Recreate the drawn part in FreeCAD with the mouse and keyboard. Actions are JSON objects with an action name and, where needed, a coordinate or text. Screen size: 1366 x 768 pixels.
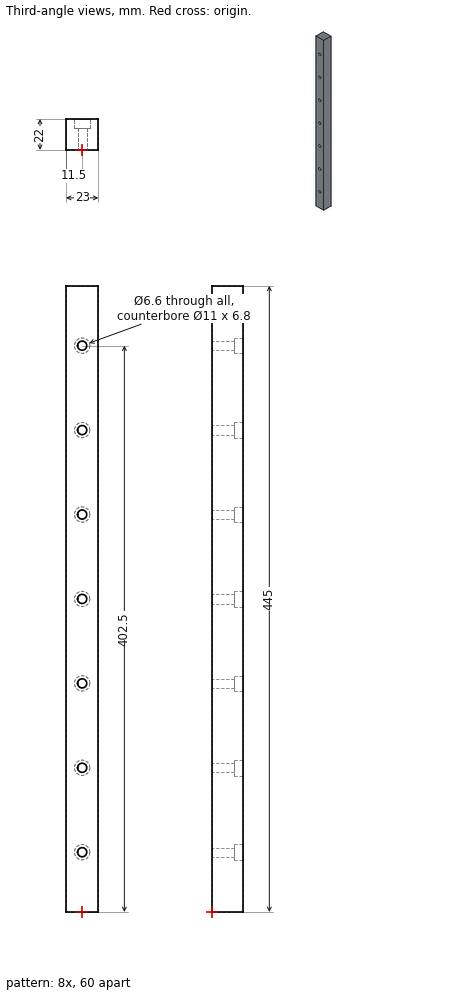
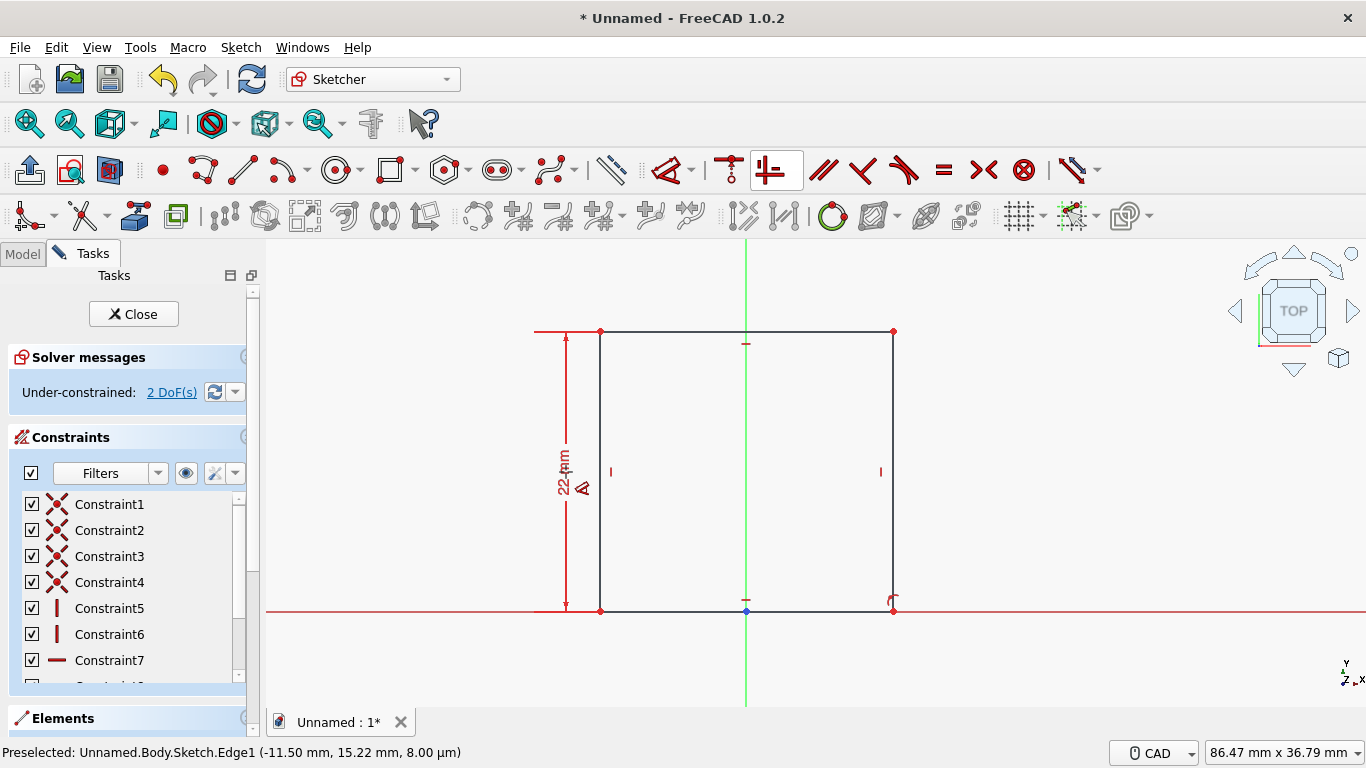
{"action": "left_click", "coordinate": [688, 612]}
{"action": "left_click", "coordinate": [679, 646]}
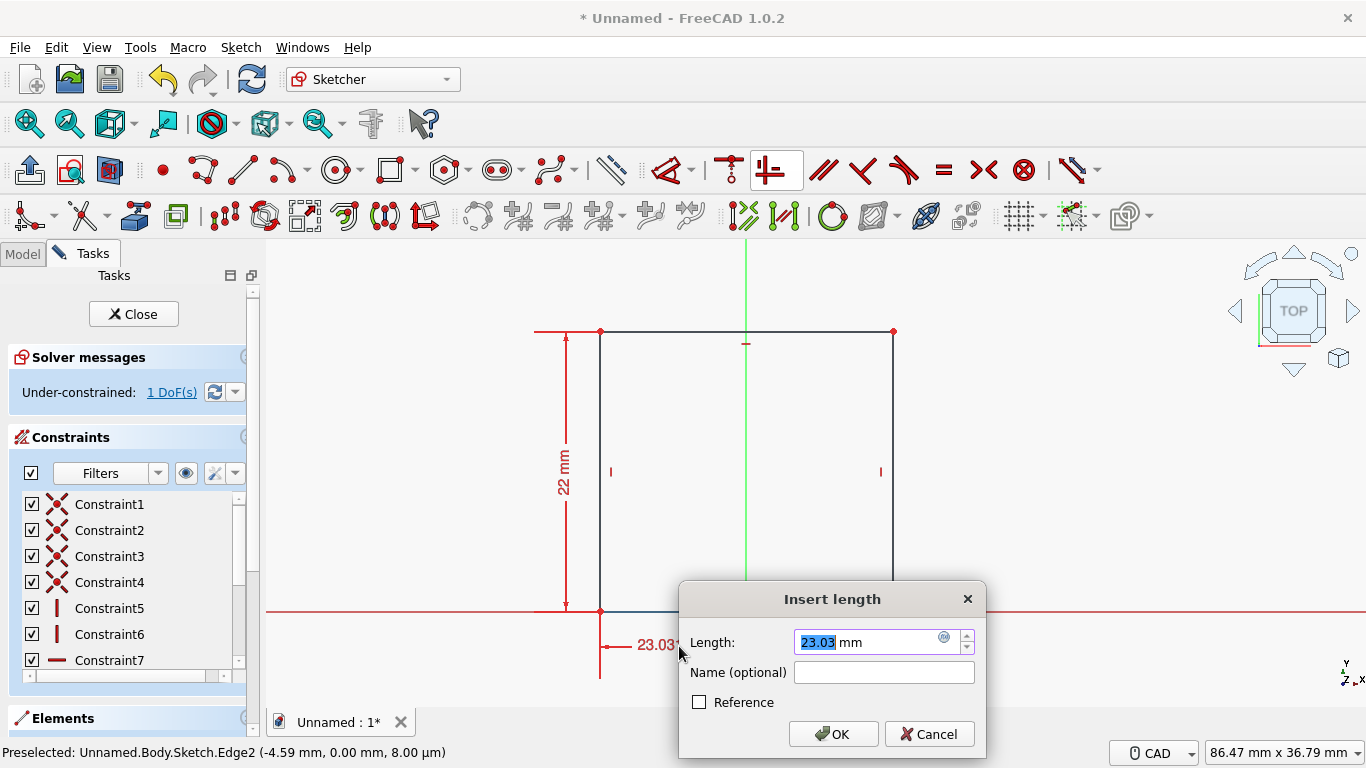
{"action": "type", "text": "23"}
{"action": "key", "text": "Return"}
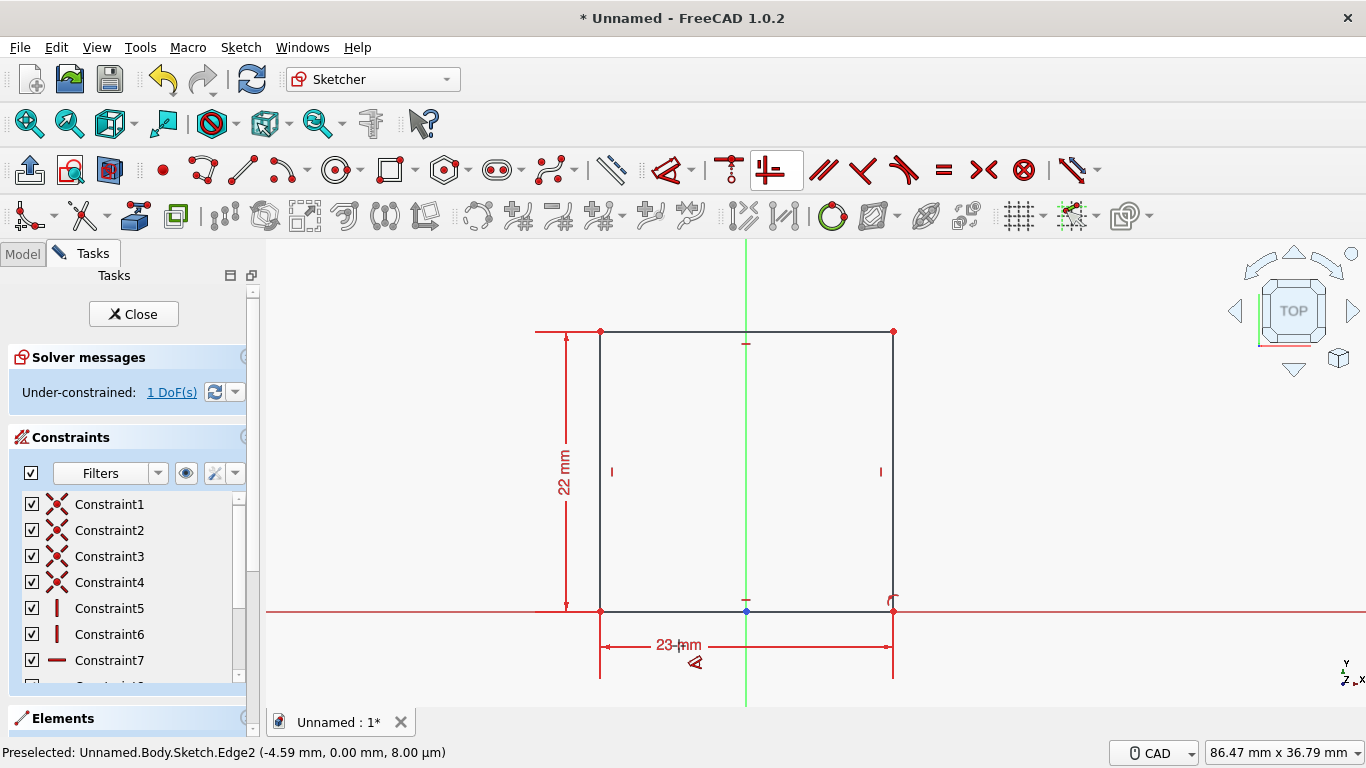
{"action": "left_click", "coordinate": [600, 332]}
{"action": "left_click", "coordinate": [673, 298]}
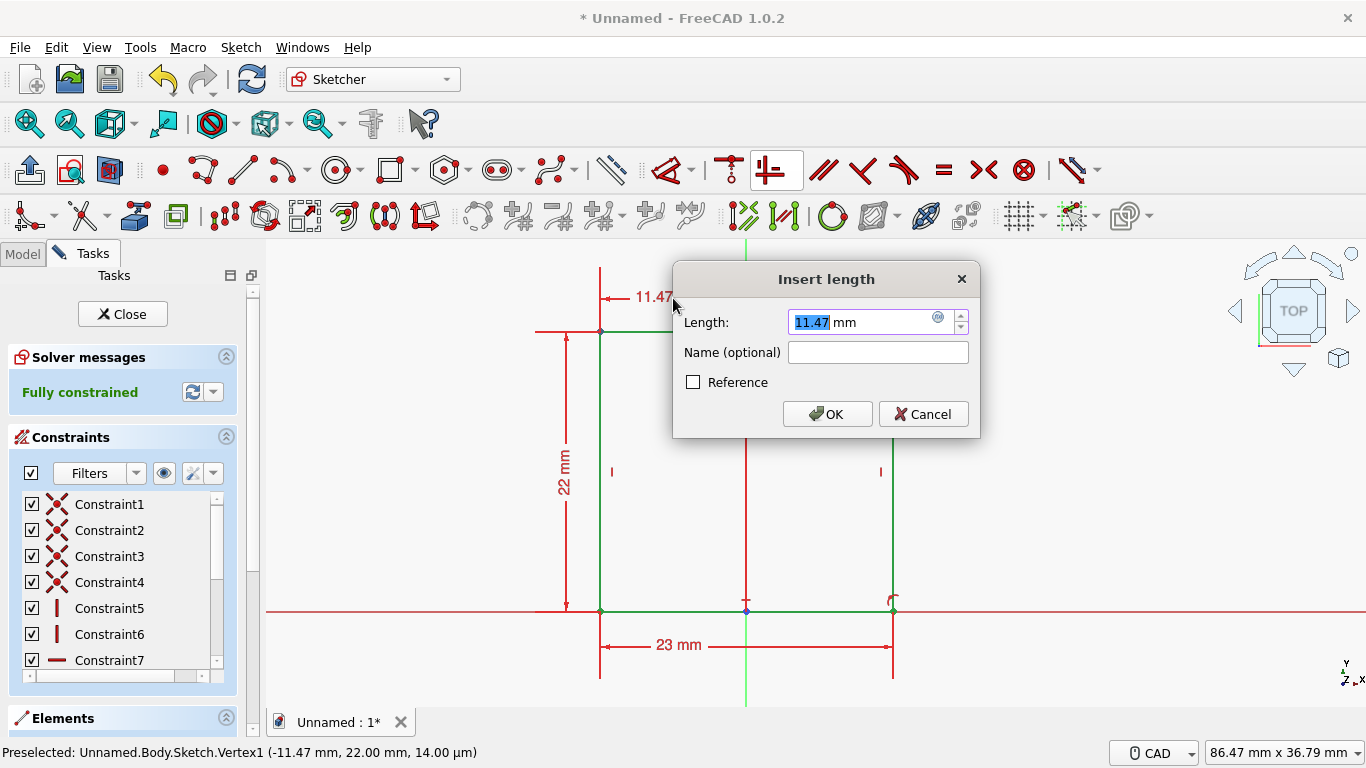
{"action": "type", "text": "11.5"}
{"action": "key", "text": "Return"}
{"action": "key", "text": "Escape"}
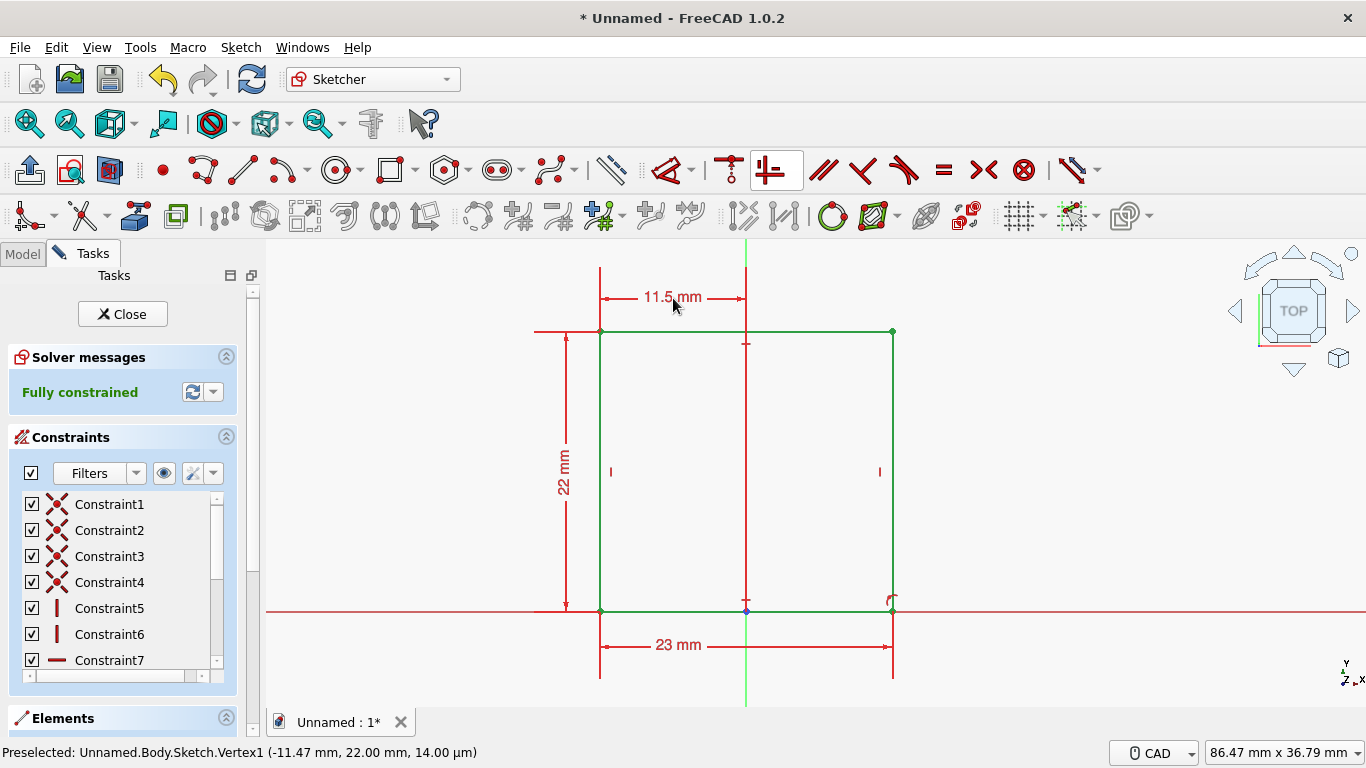
{"action": "left_click", "coordinate": [123, 314]}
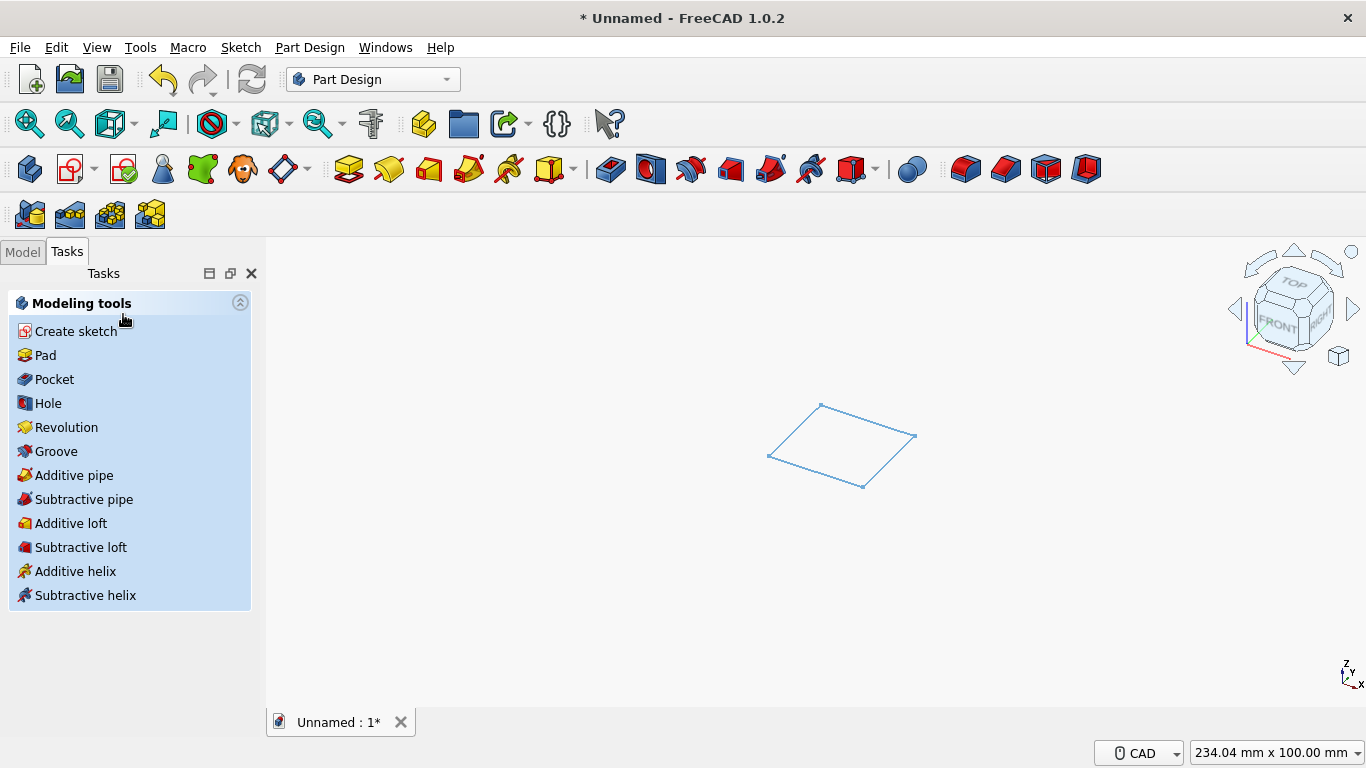
{"action": "left_click", "coordinate": [350, 170]}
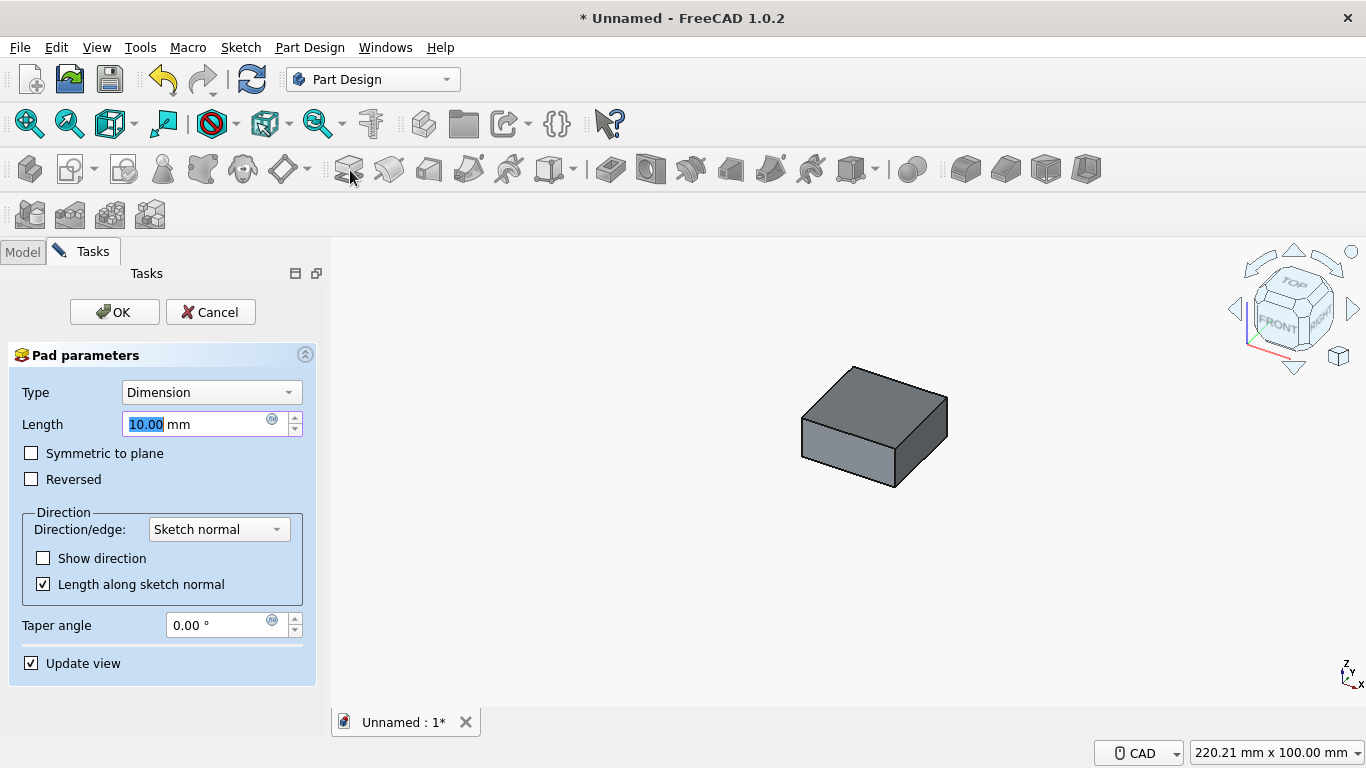
{"action": "type", "text": "445"}
{"action": "key", "text": "Tab"}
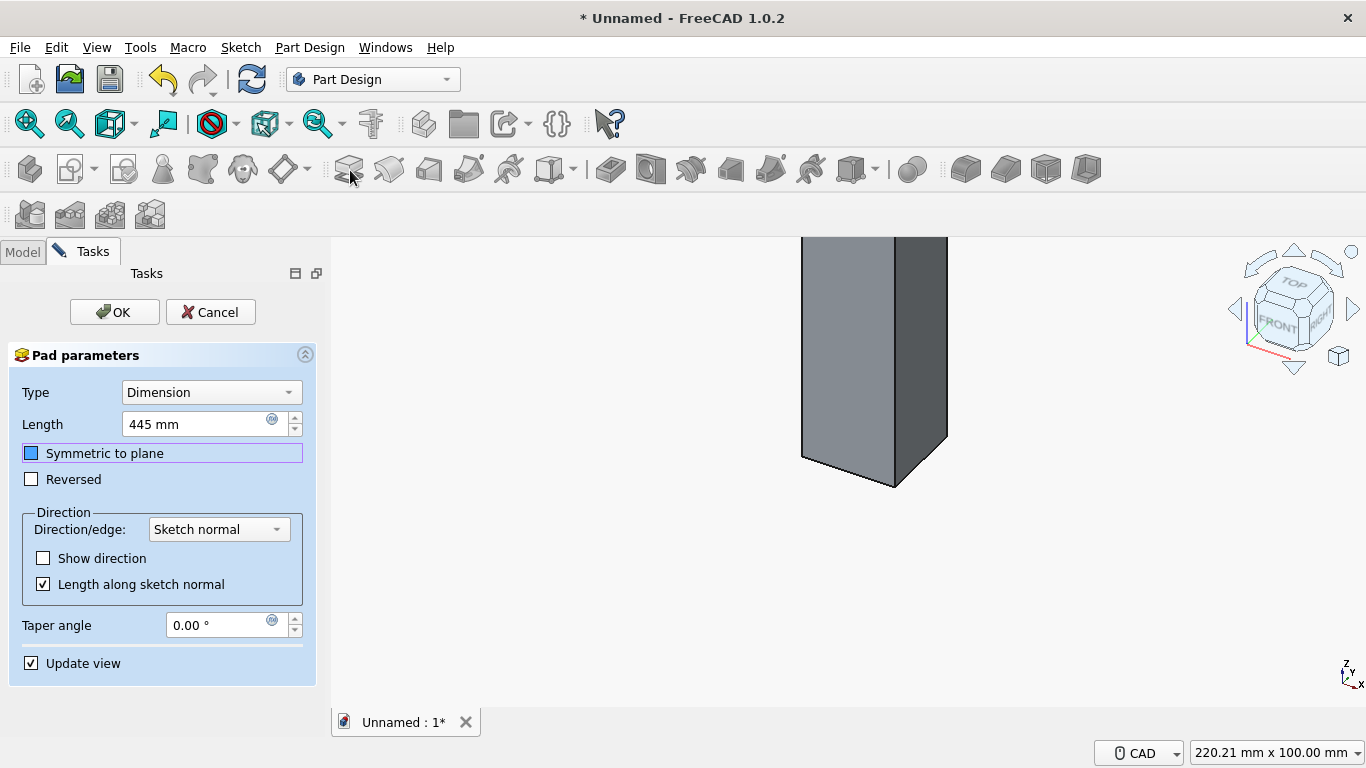
{"action": "left_click", "coordinate": [115, 312]}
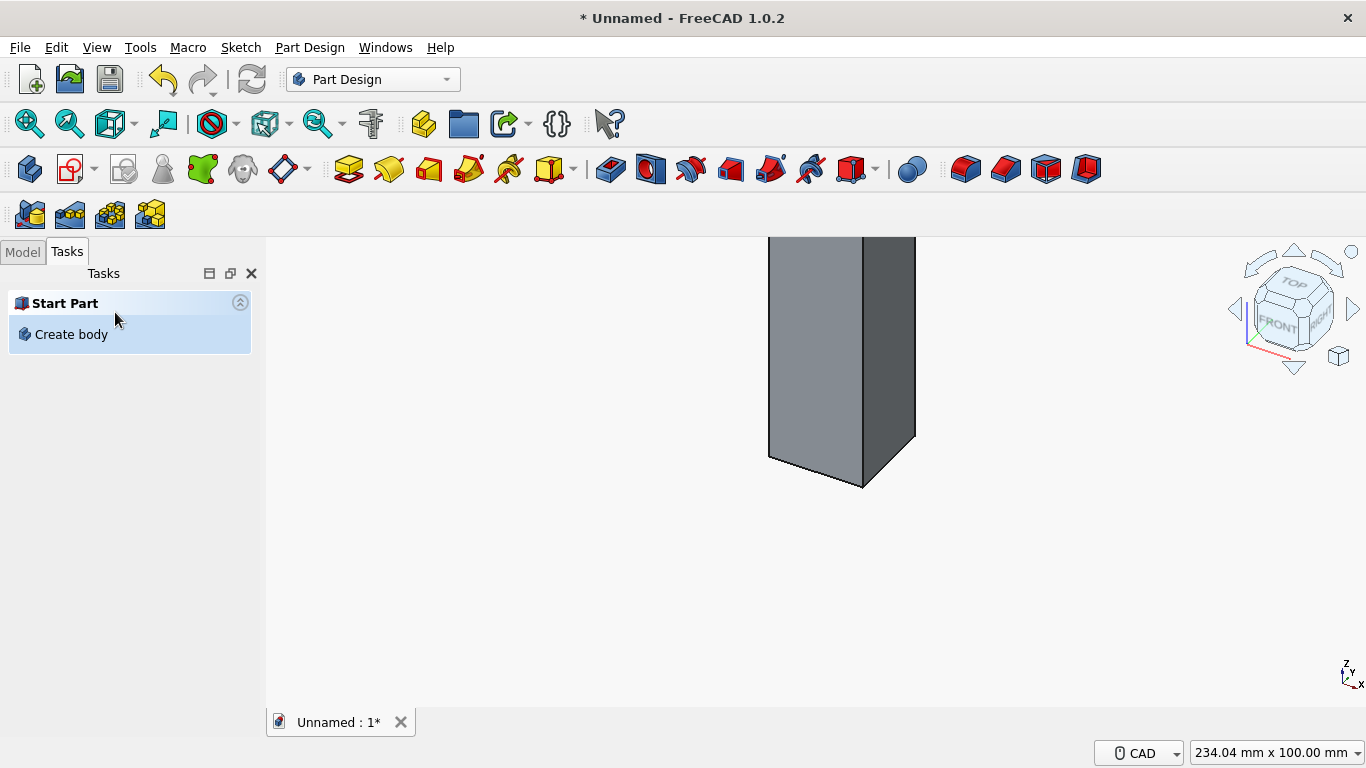
{"action": "key", "text": "v f"}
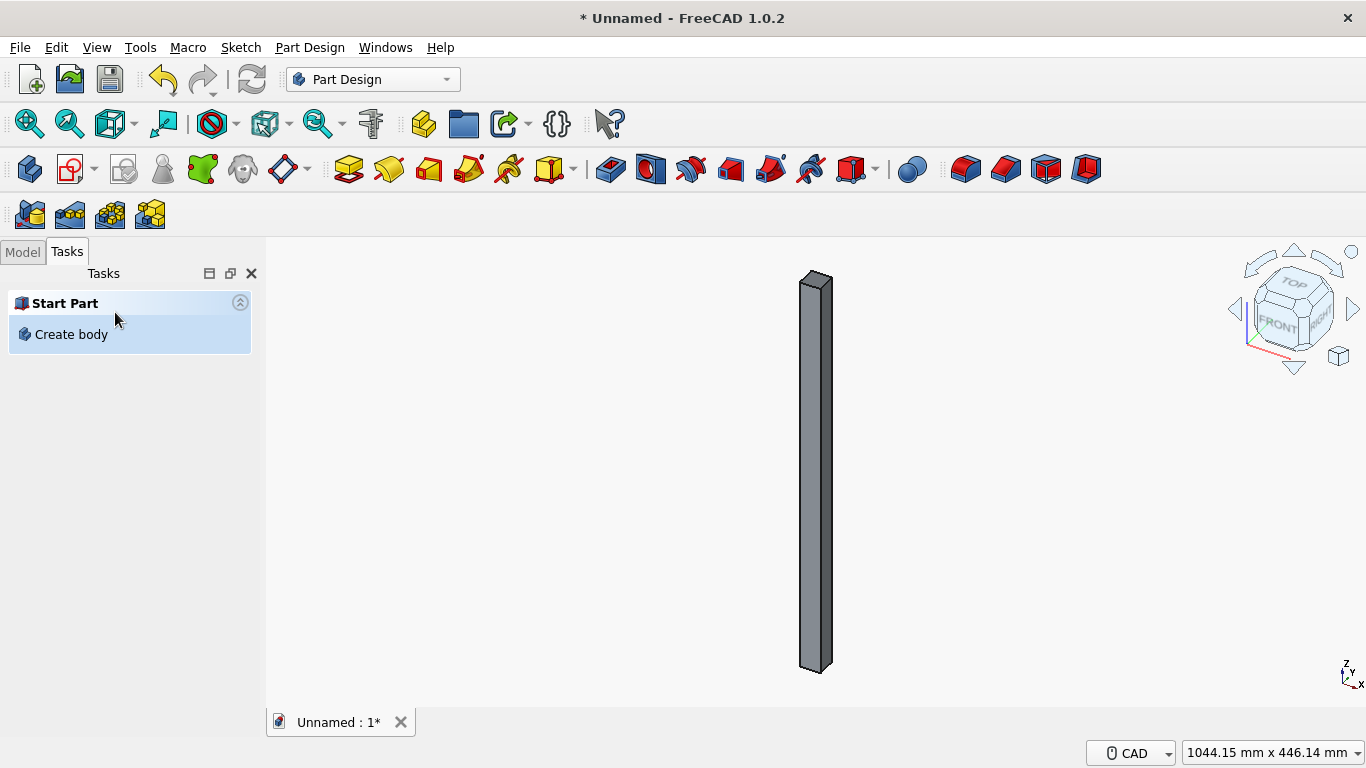
{"action": "key", "text": "4"}